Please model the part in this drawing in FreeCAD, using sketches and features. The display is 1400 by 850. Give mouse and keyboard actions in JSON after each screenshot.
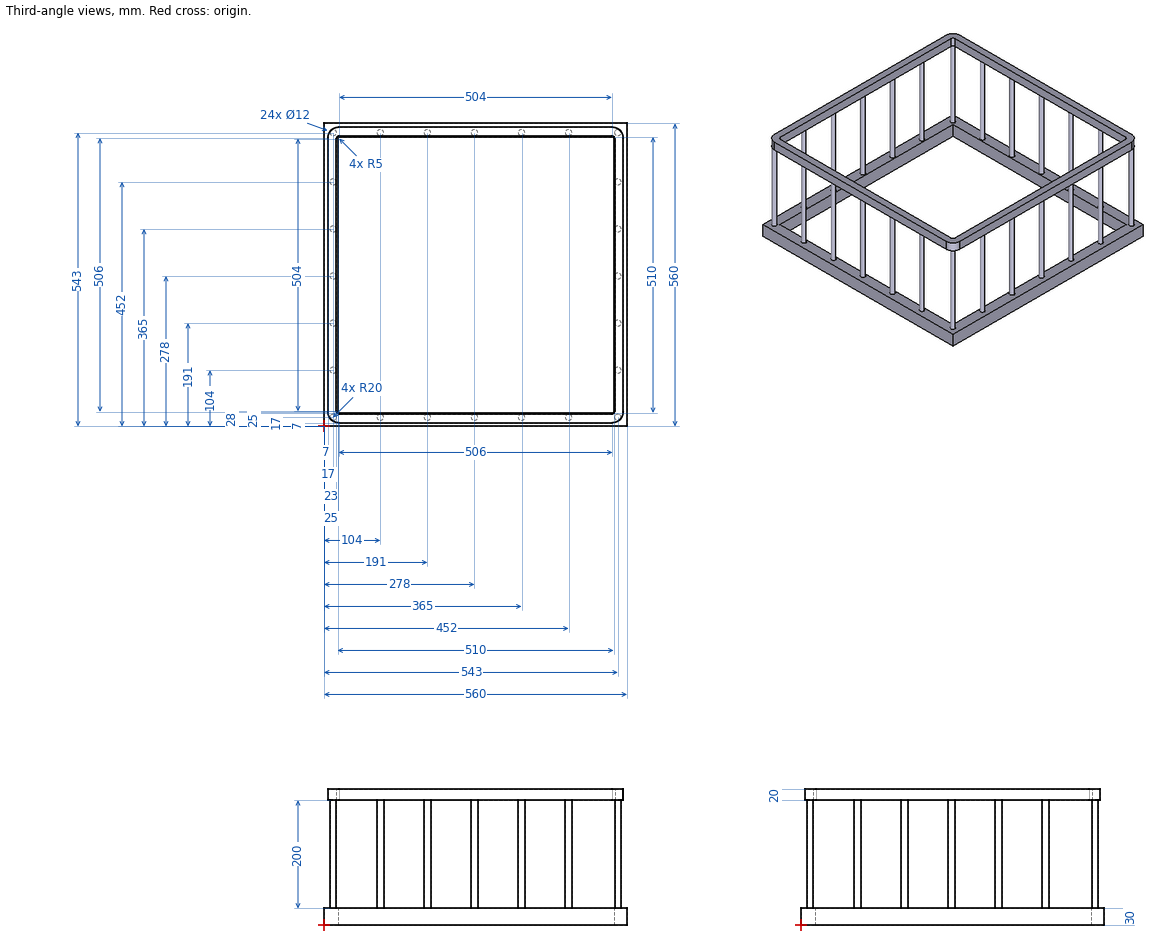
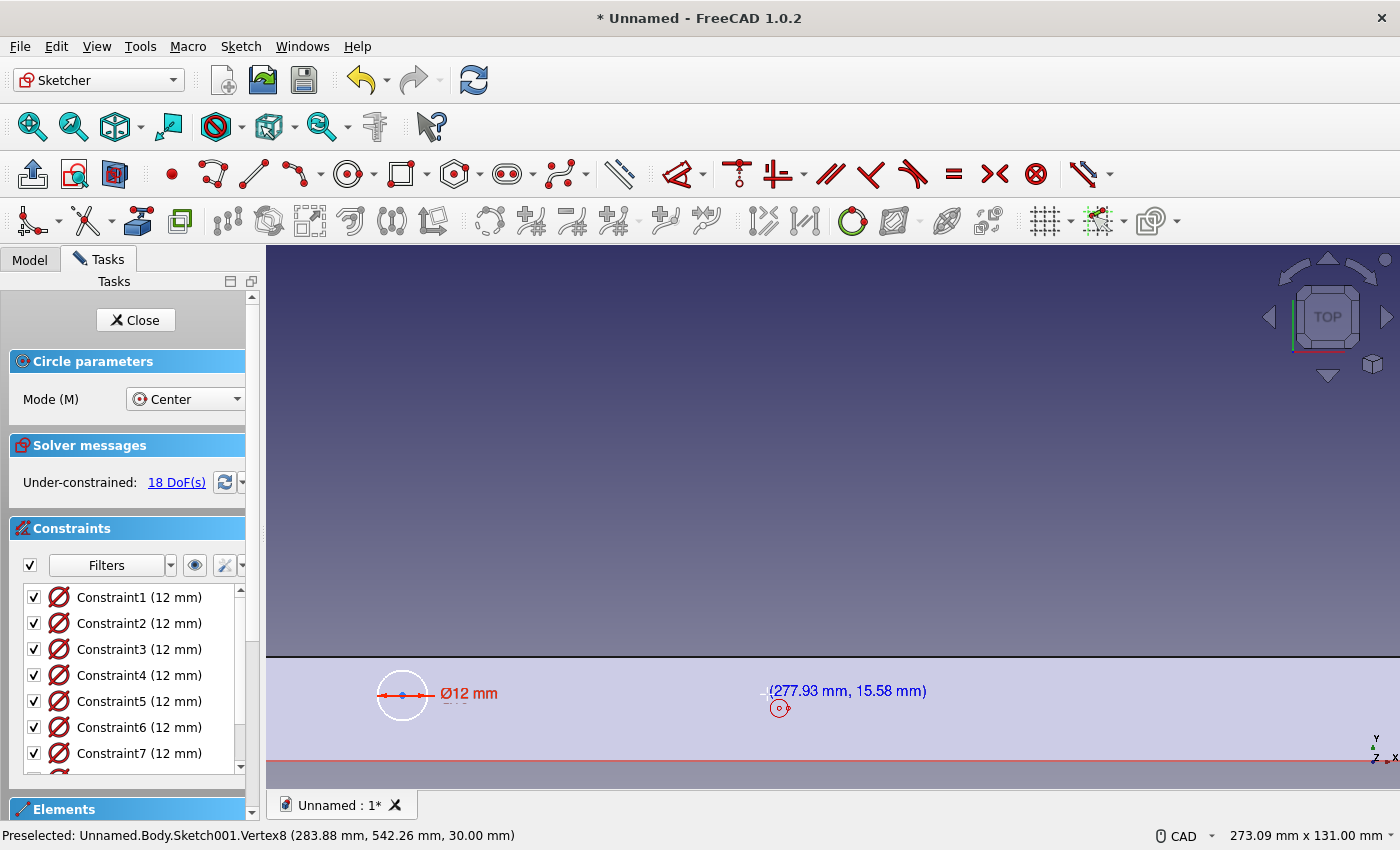
{"action": "scroll", "coordinate": [767, 694], "scroll_direction": "down", "scroll_amount": 9}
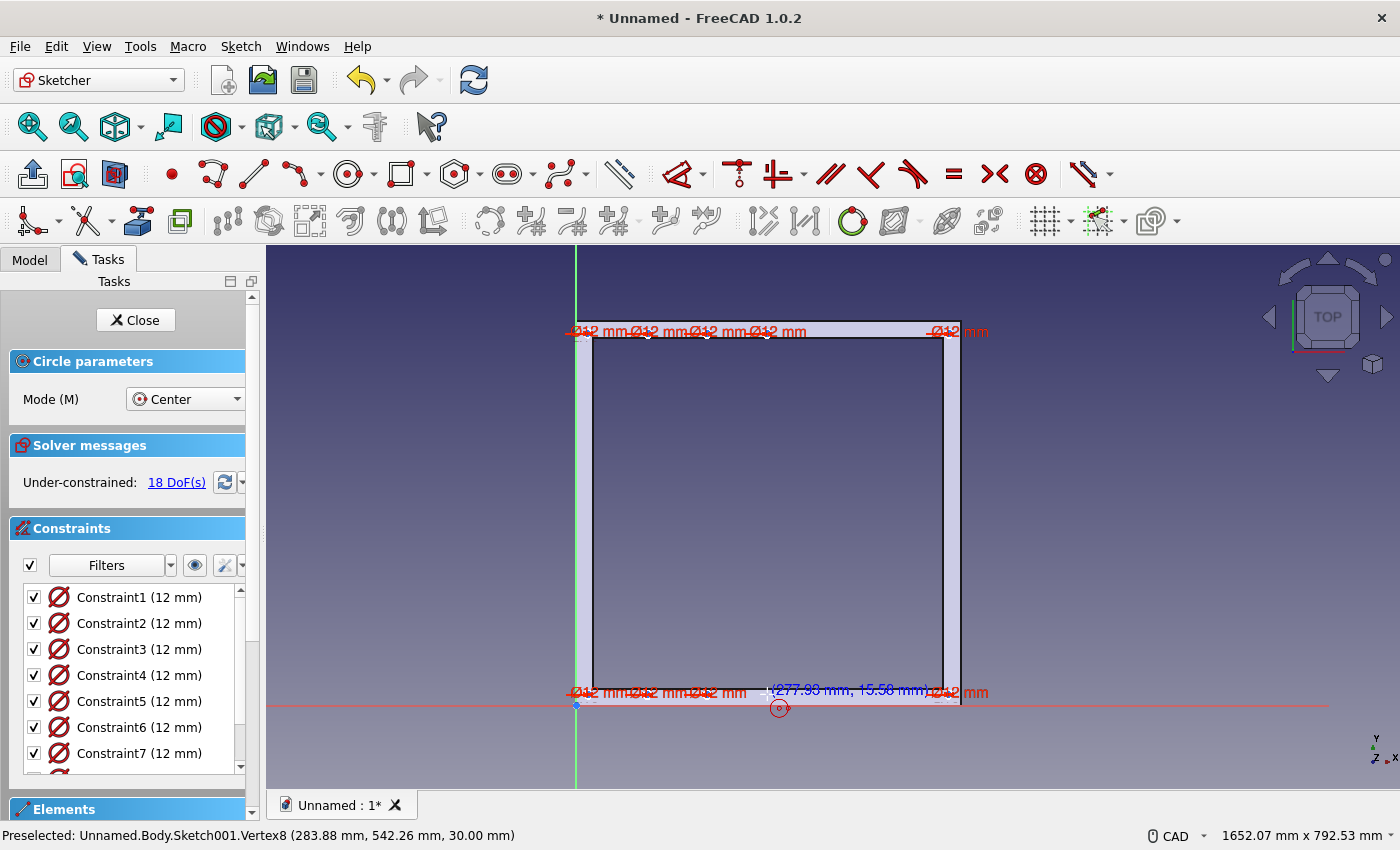
{"action": "scroll", "coordinate": [767, 694], "scroll_direction": "up", "scroll_amount": 2}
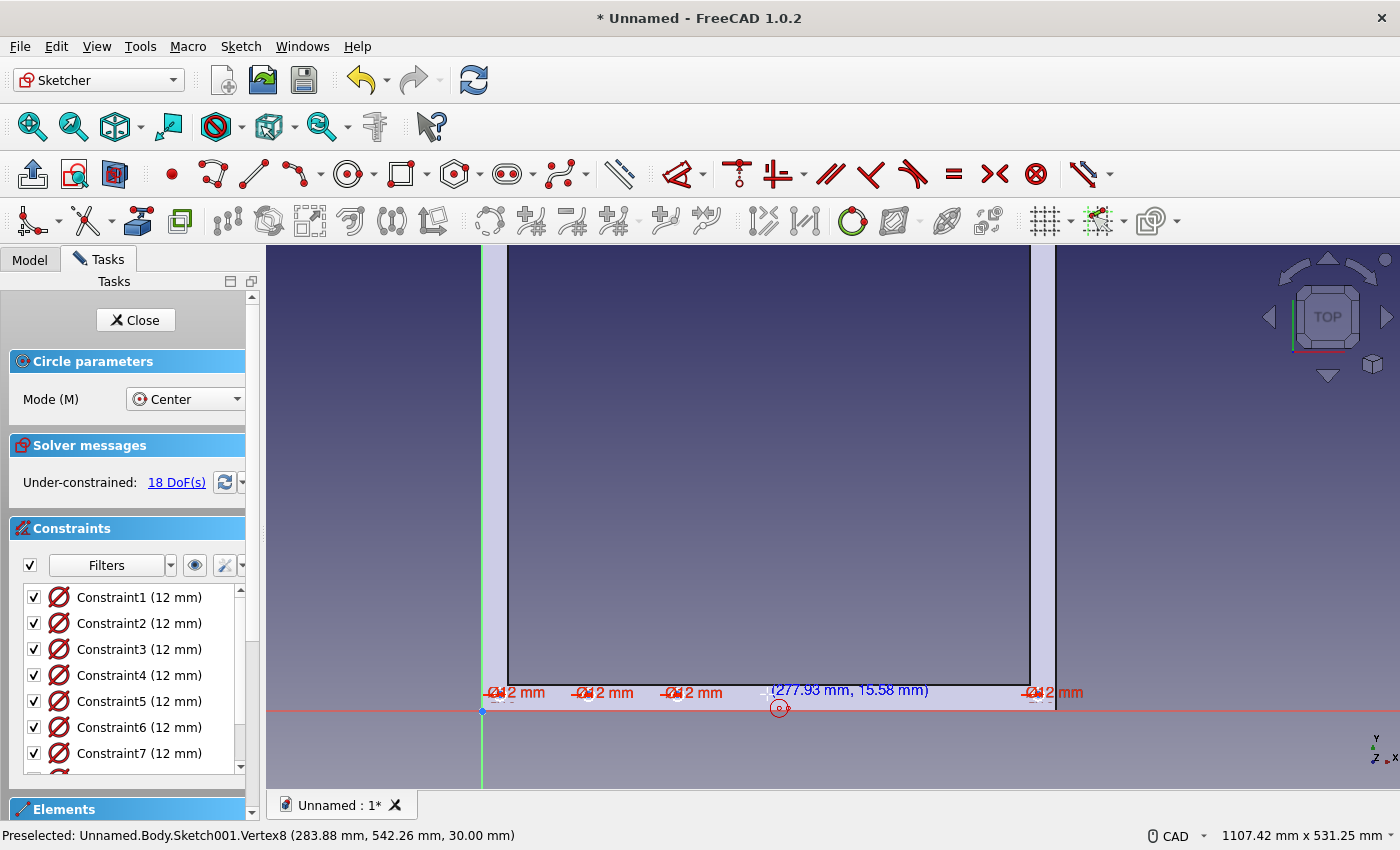
{"action": "left_click", "coordinate": [767, 694]}
{"action": "mouse_move", "coordinate": [771, 689]}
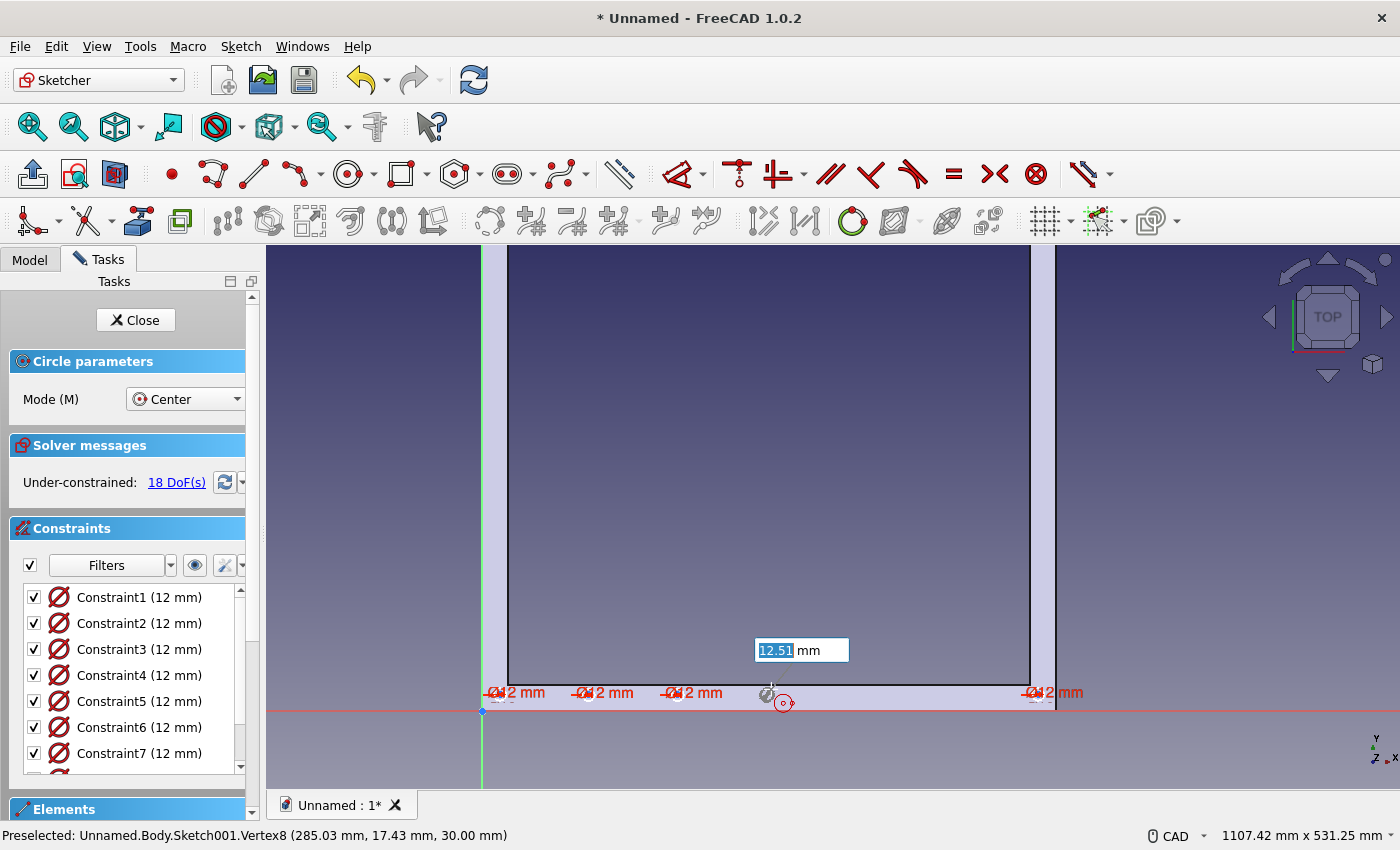
{"action": "type", "text": "12"}
{"action": "key", "text": "Return"}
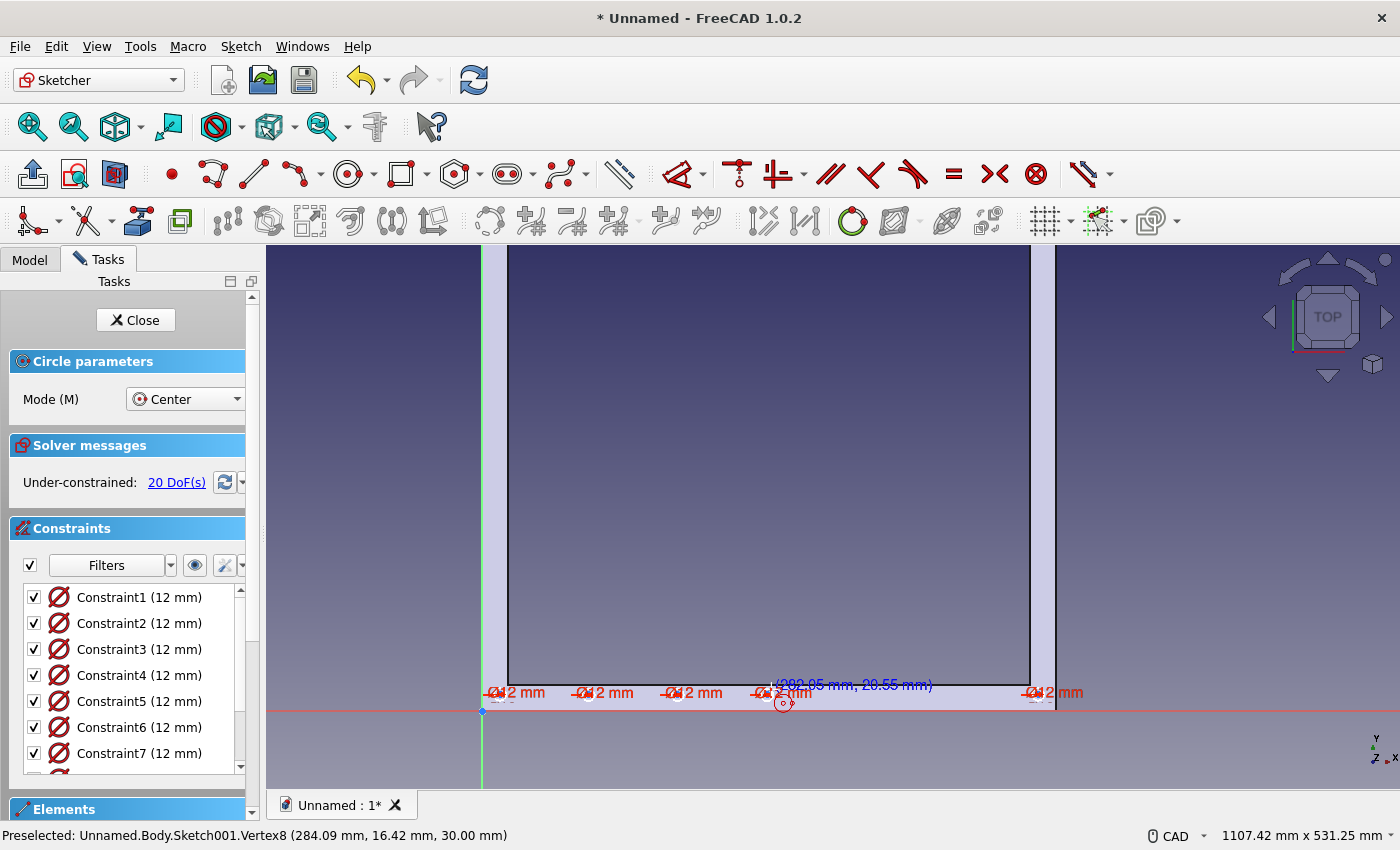
{"action": "scroll", "coordinate": [767, 694], "scroll_direction": "down", "scroll_amount": 2}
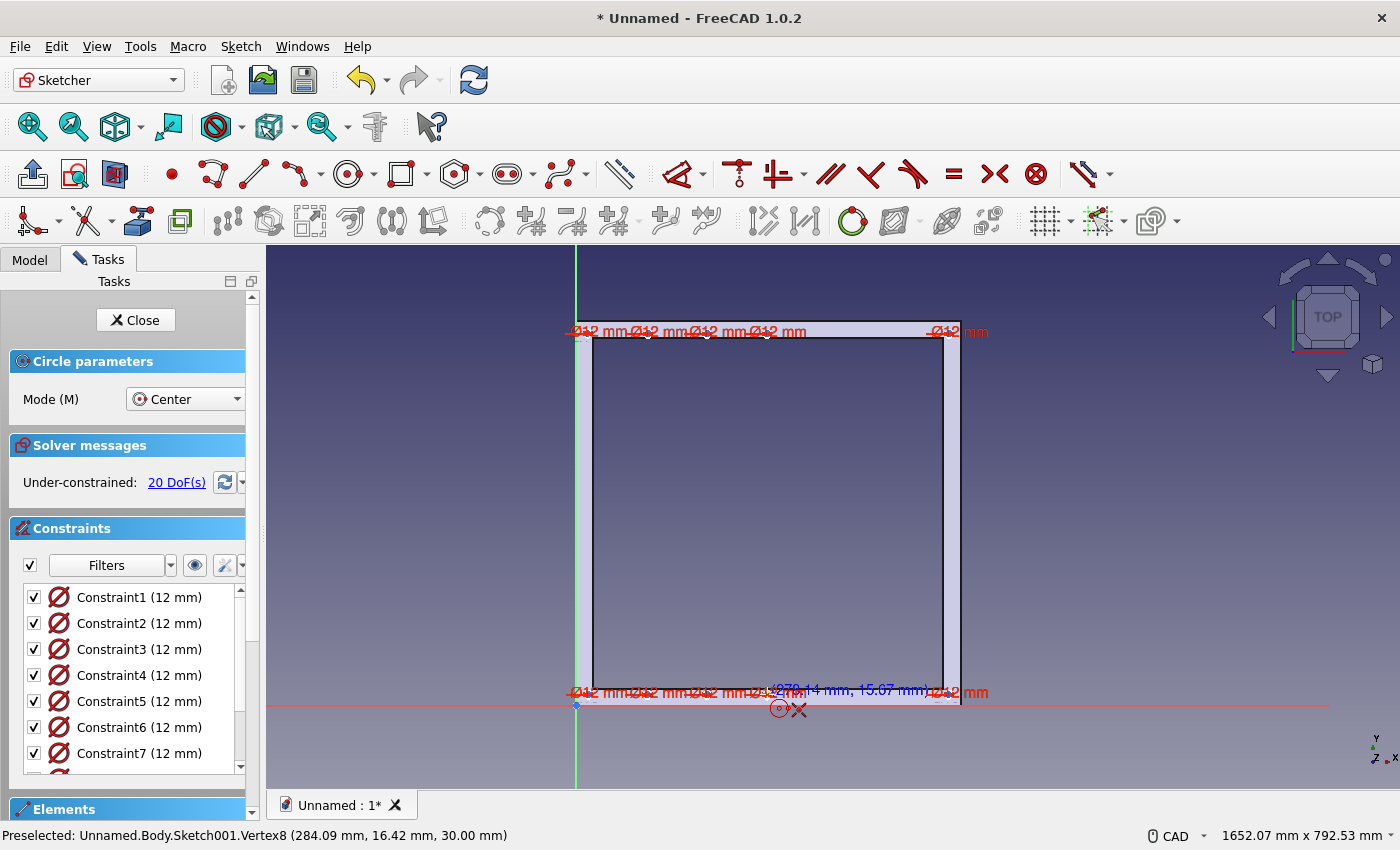
{"action": "scroll", "coordinate": [827, 333], "scroll_direction": "up", "scroll_amount": 9}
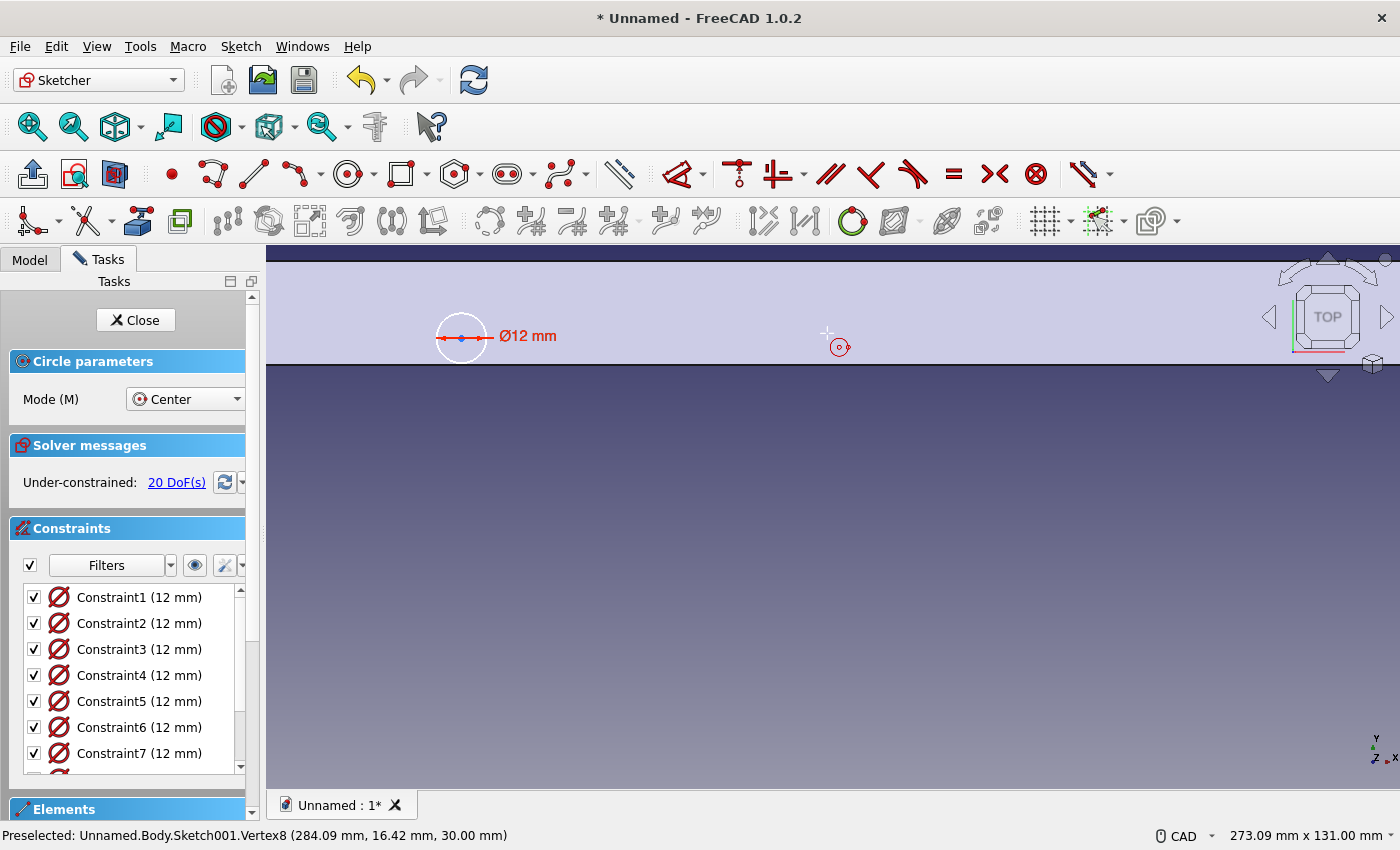
{"action": "scroll", "coordinate": [827, 333], "scroll_direction": "down", "scroll_amount": 9}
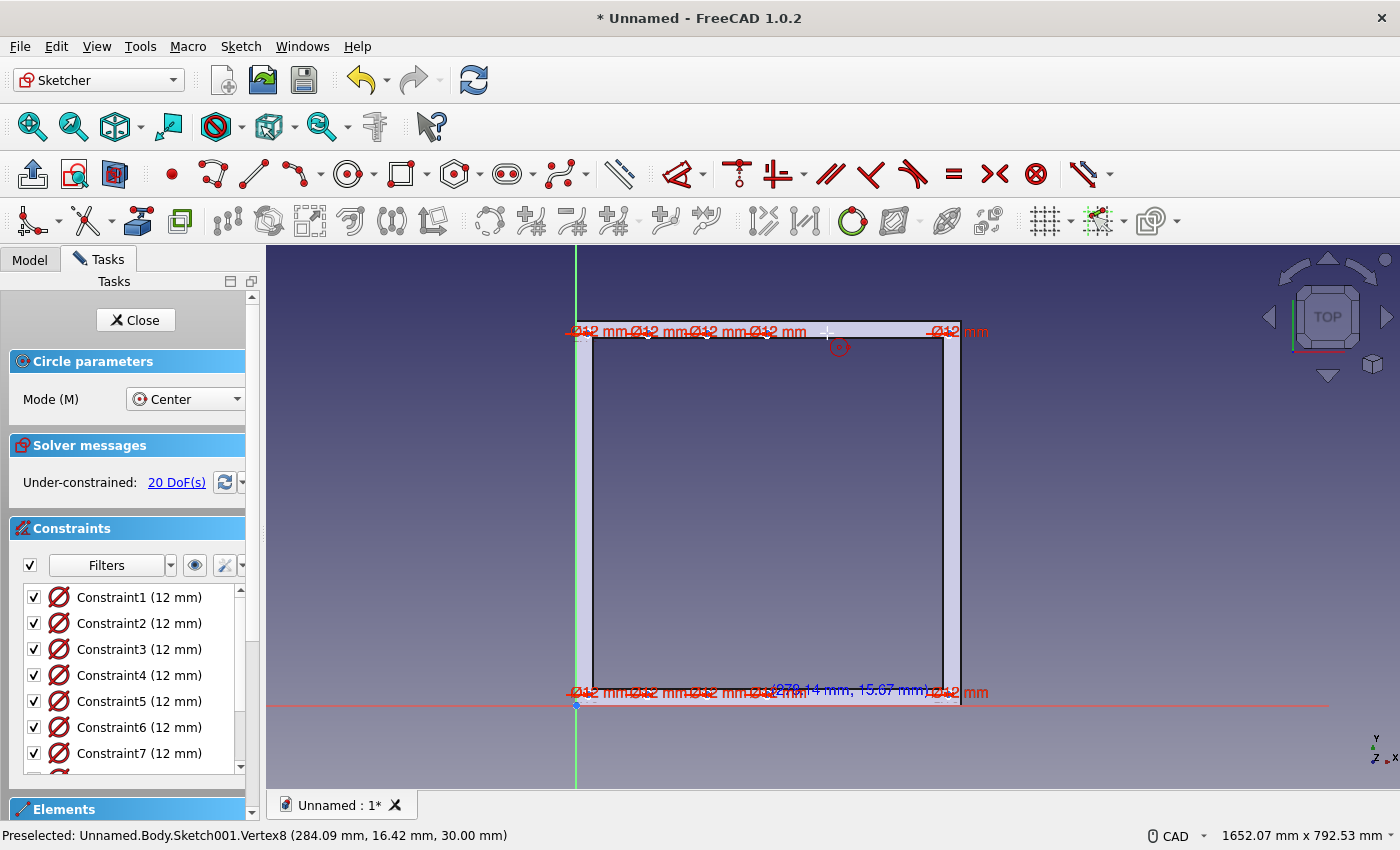
{"action": "left_click", "coordinate": [827, 333]}
{"action": "mouse_move", "coordinate": [830, 330]}